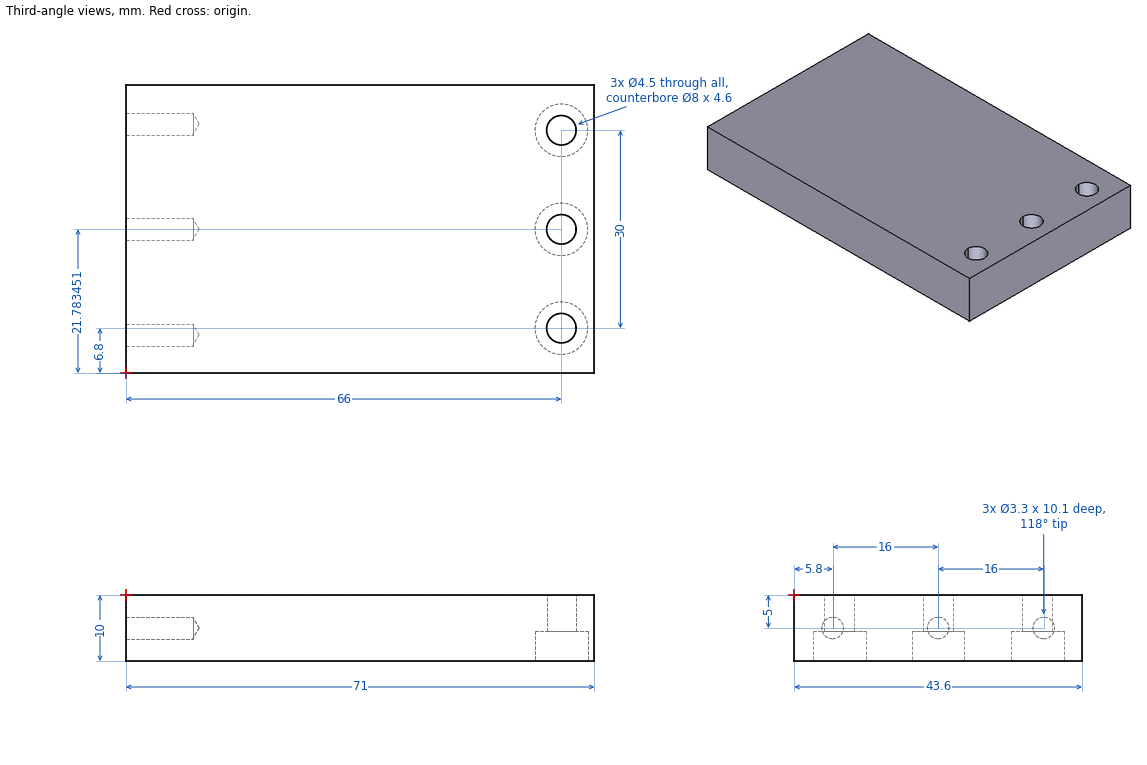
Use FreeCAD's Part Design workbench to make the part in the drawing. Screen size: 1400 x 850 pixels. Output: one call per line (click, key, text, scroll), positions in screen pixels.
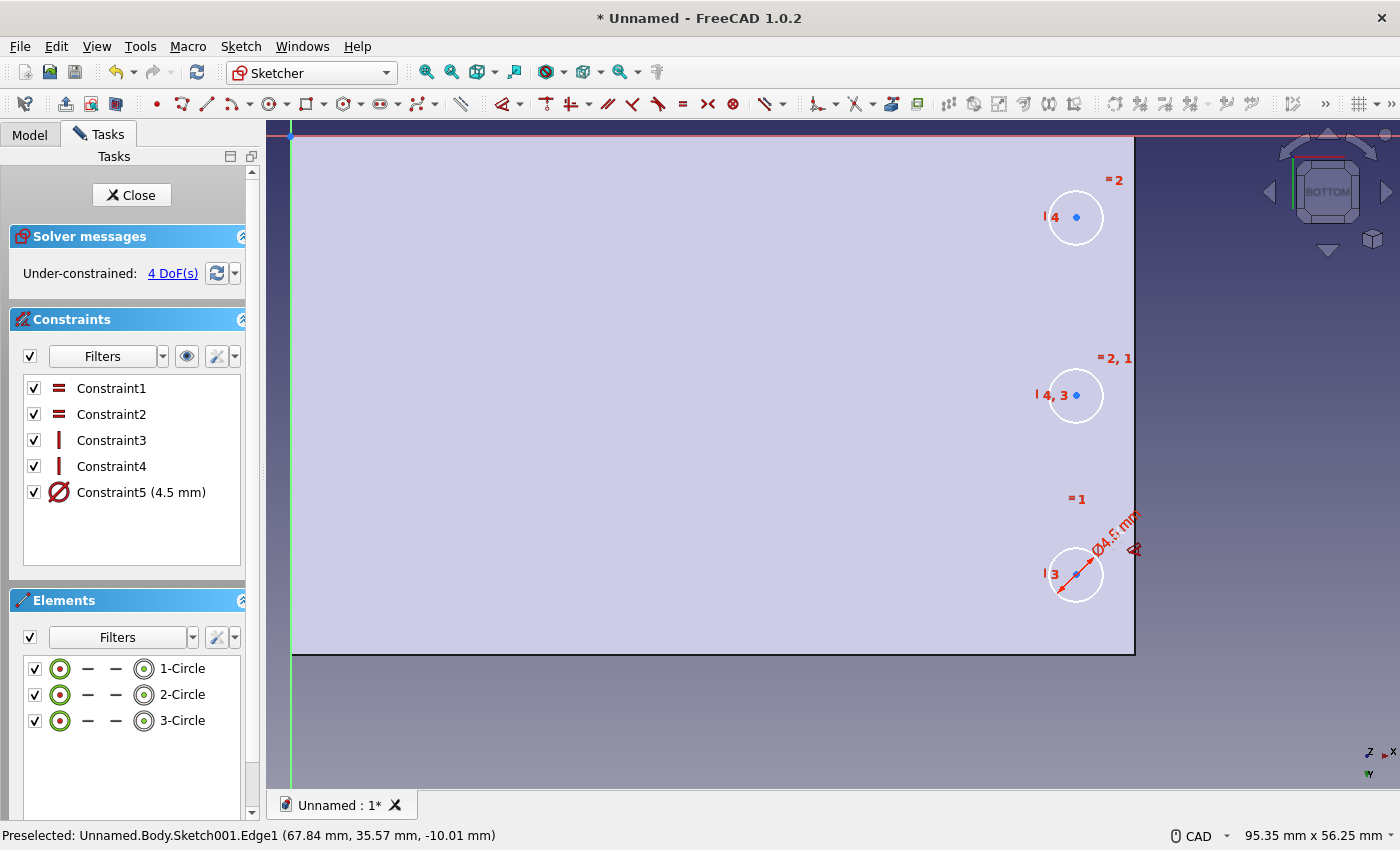
click(1076, 575)
click(685, 609)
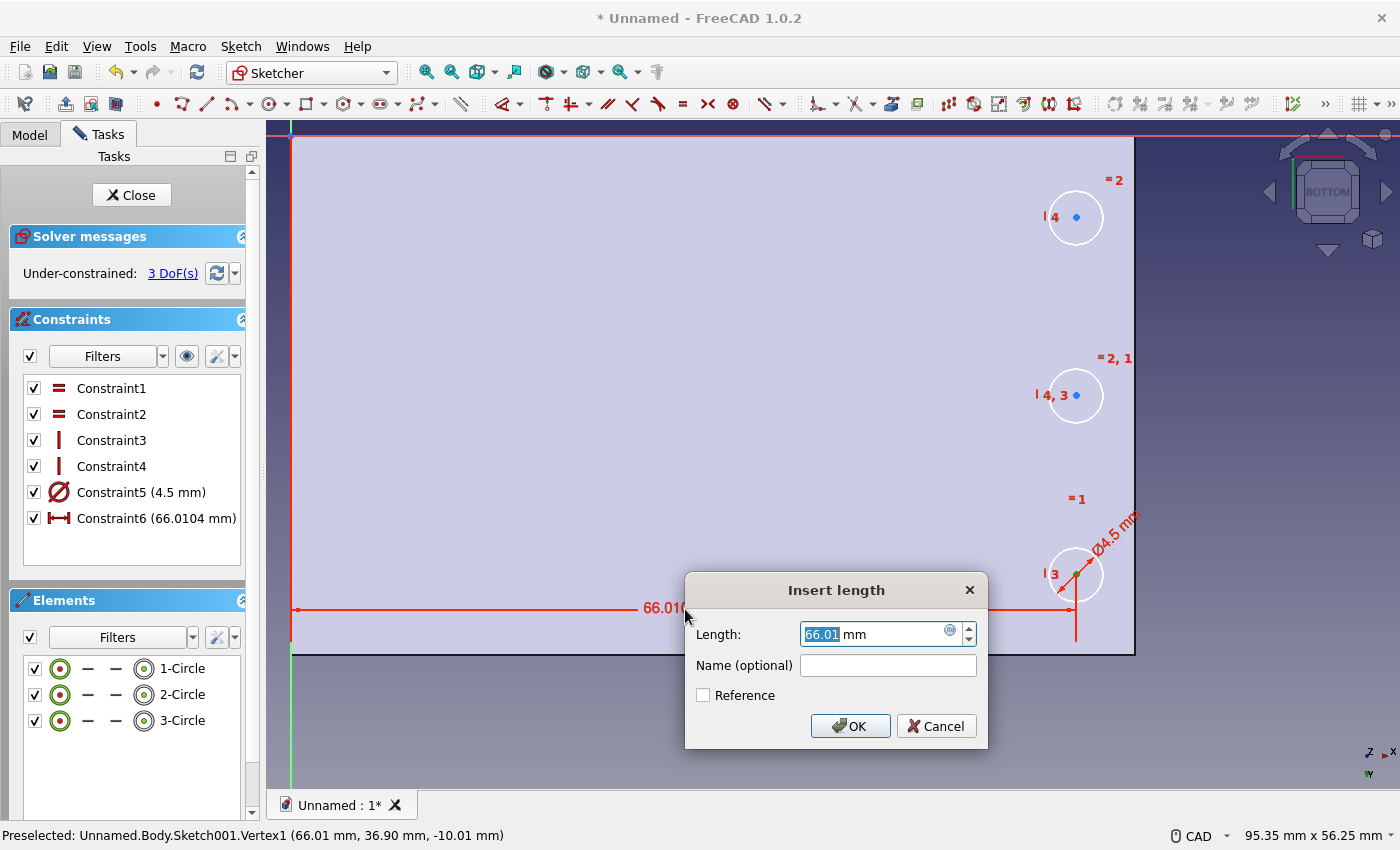
text(66)
key(Return)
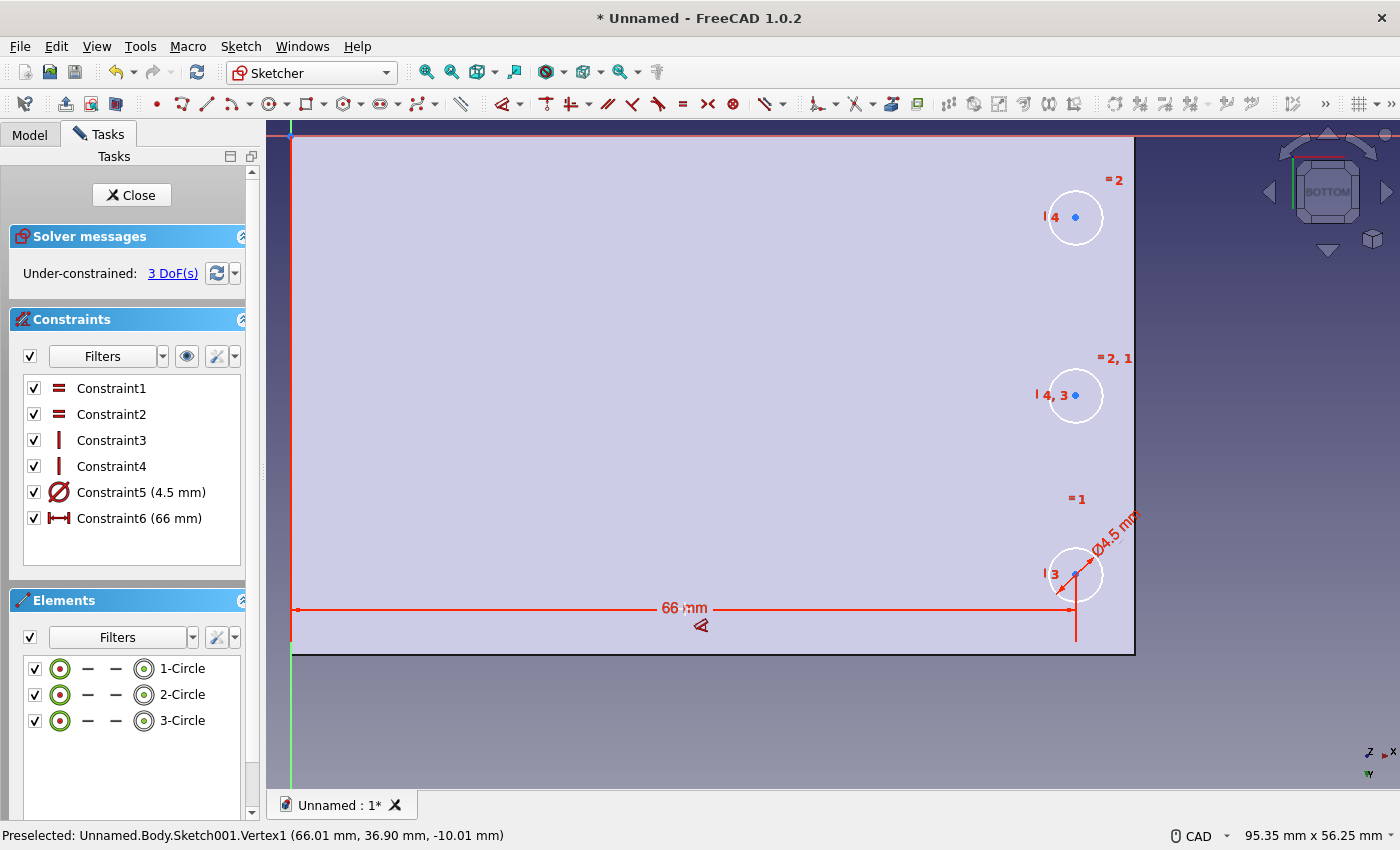
click(1076, 218)
click(1110, 183)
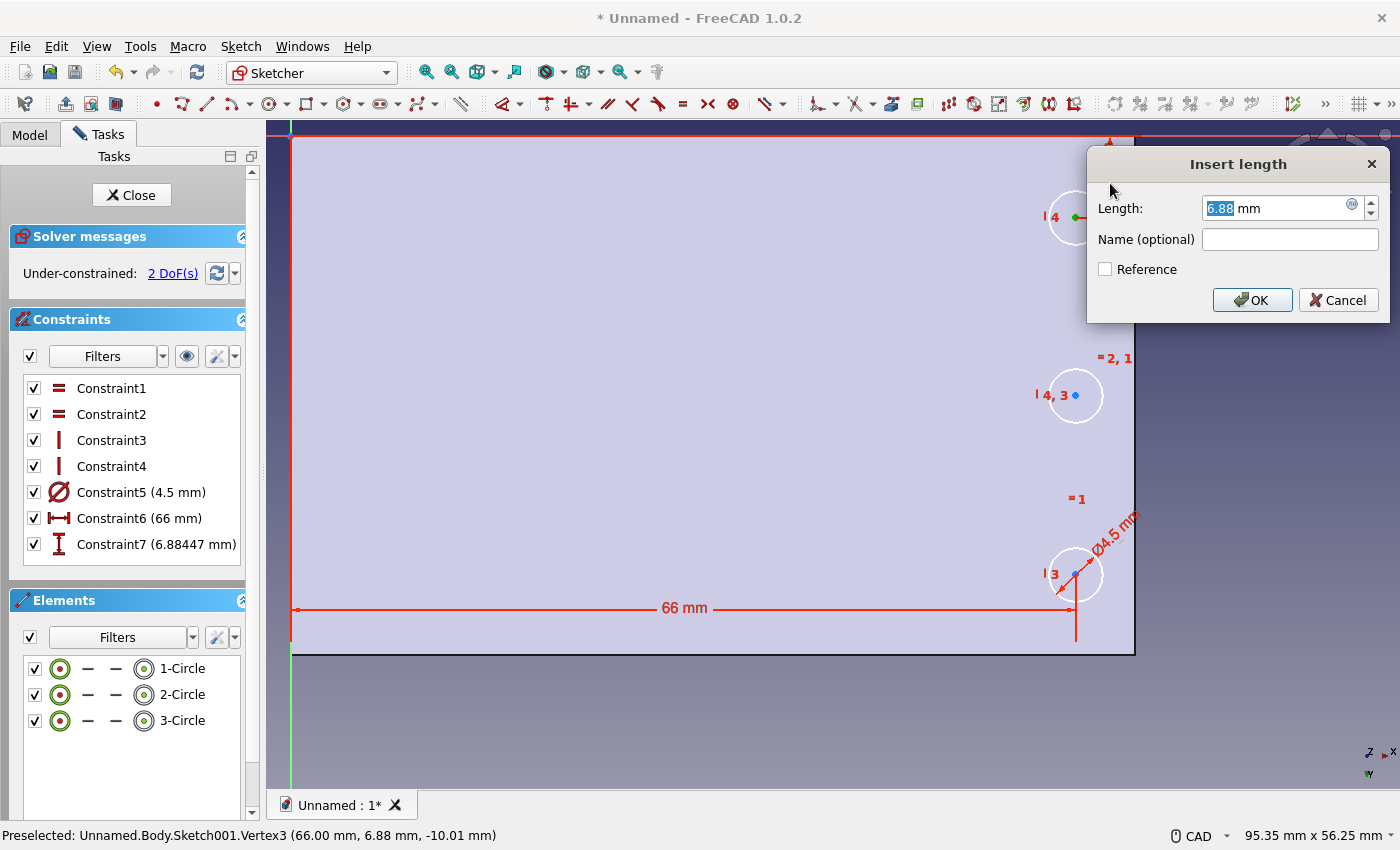
text(6.8)
key(Return)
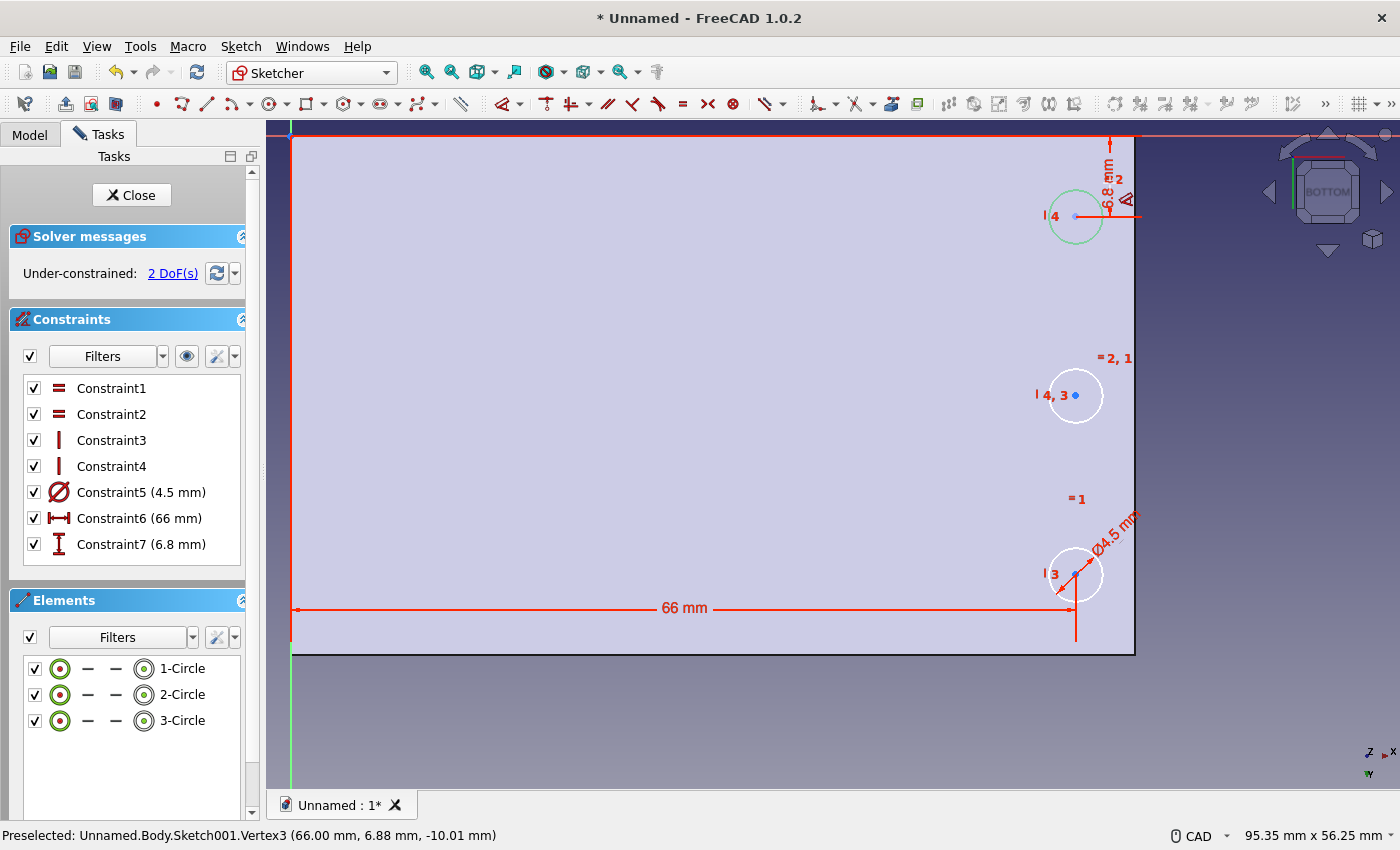
click(1076, 575)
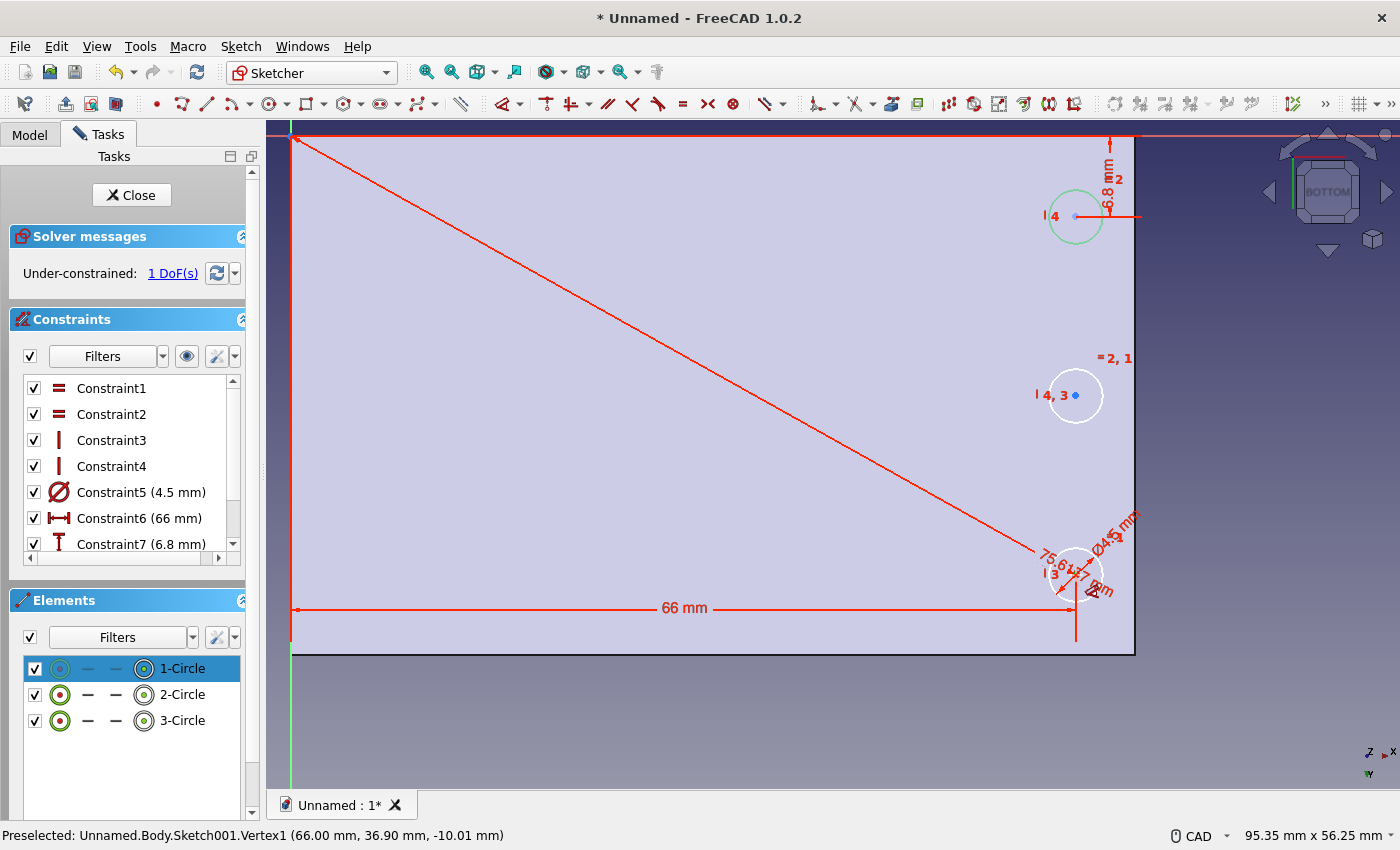
click(1076, 217)
click(1110, 314)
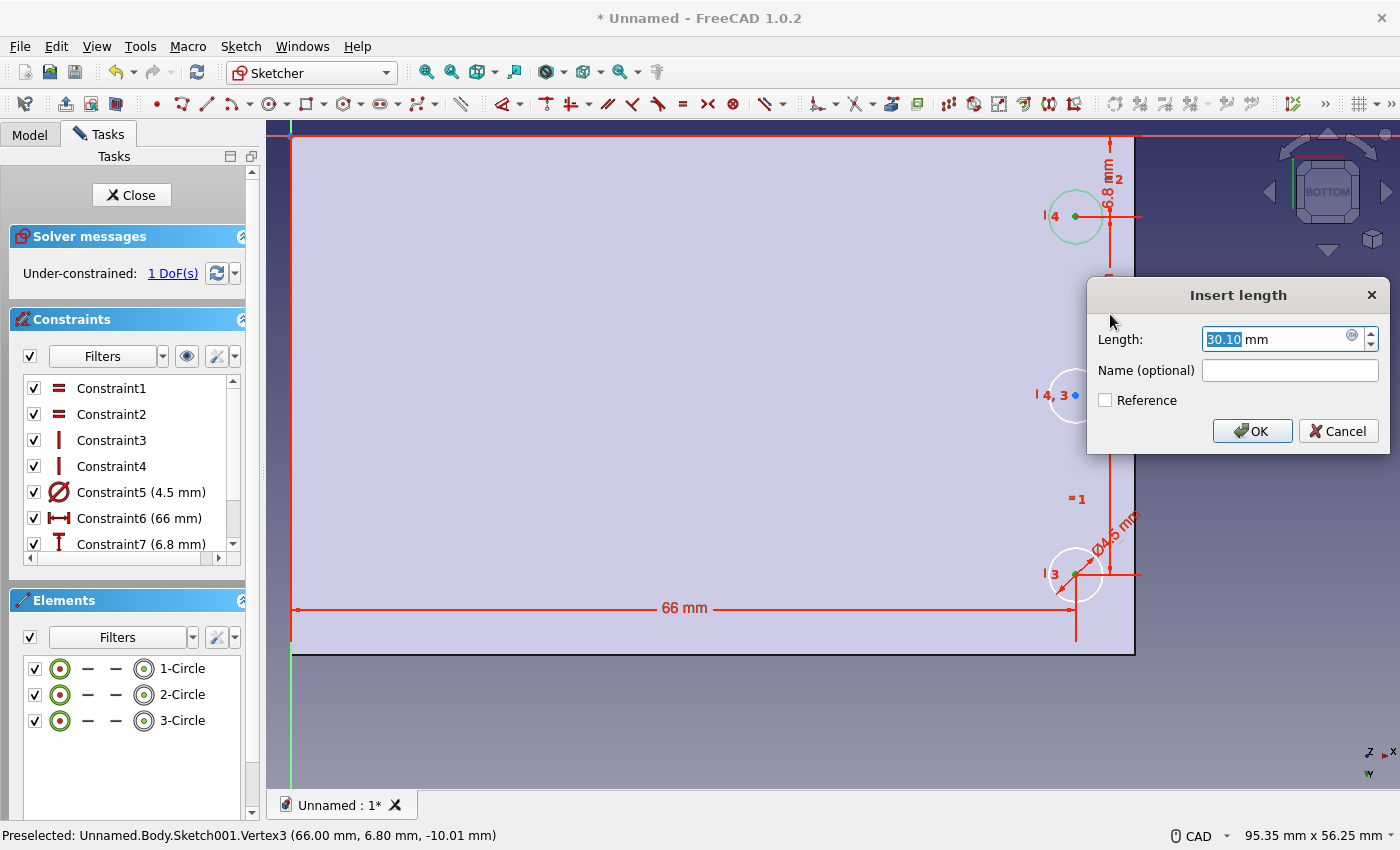
text(30)
key(Return)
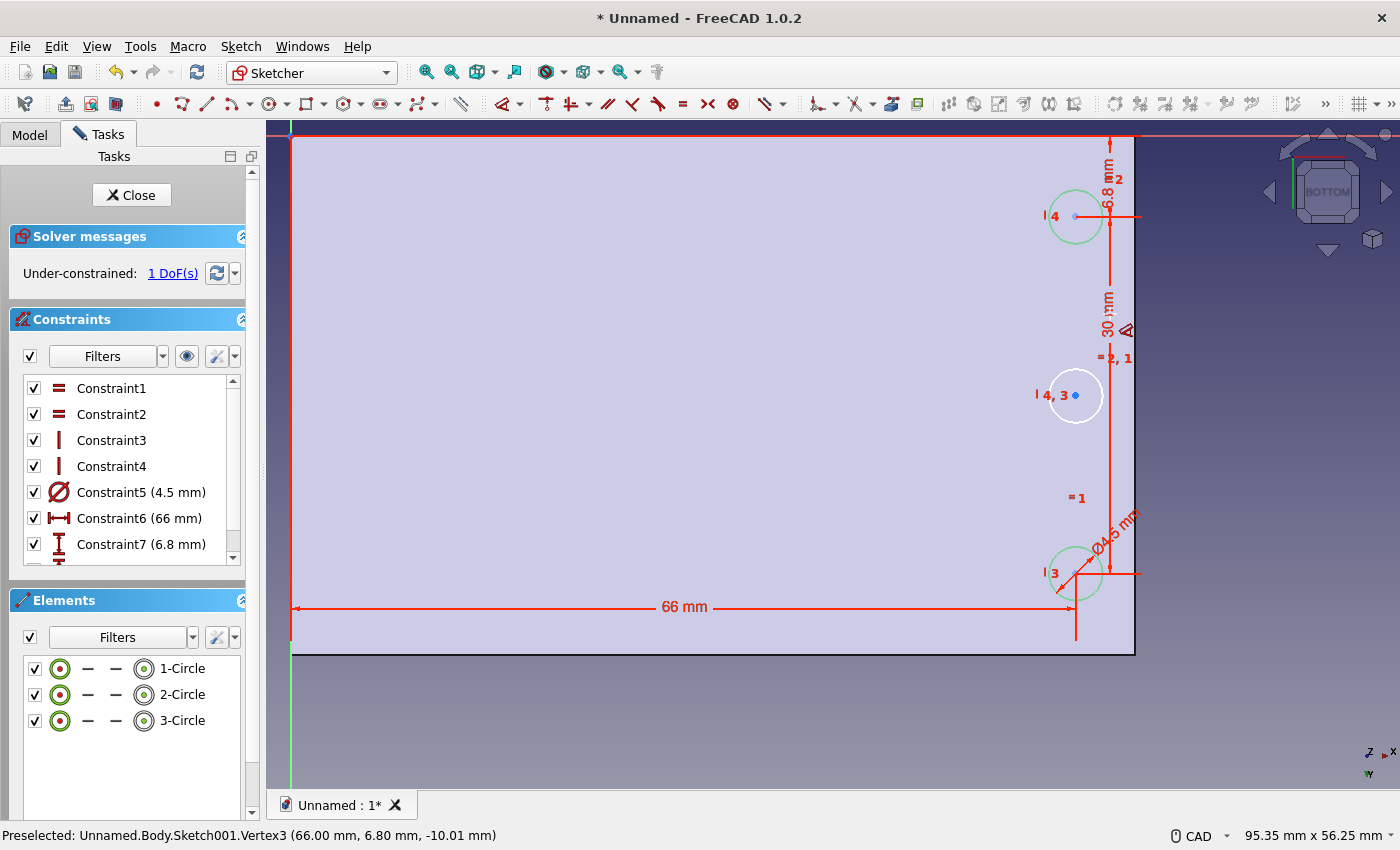
click(1076, 396)
click(1110, 272)